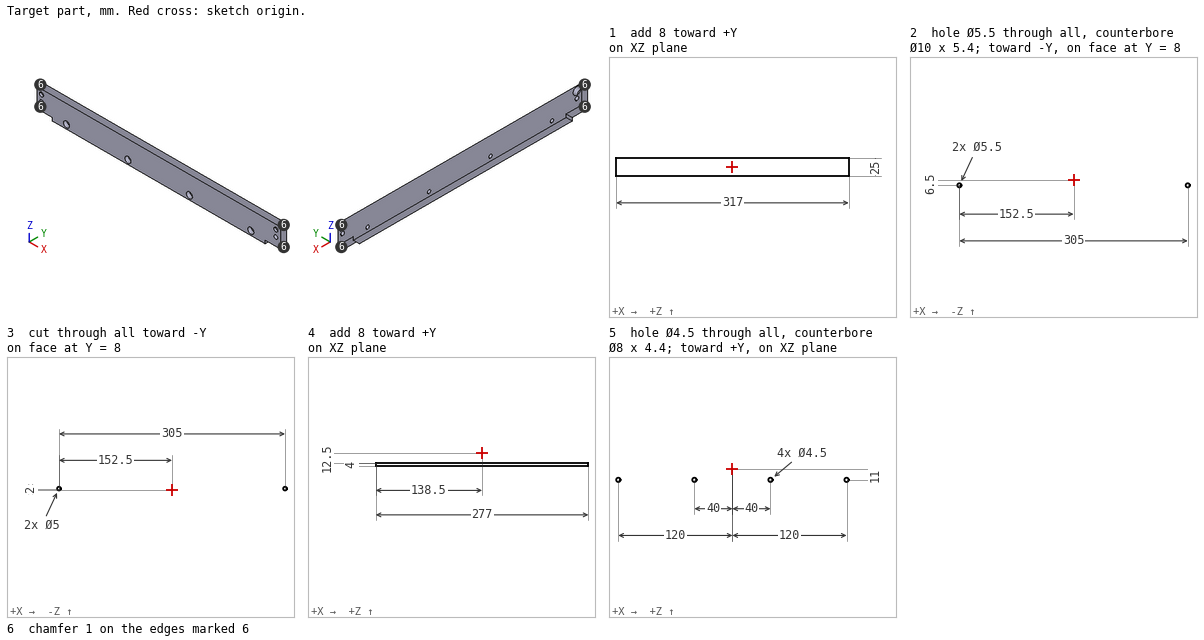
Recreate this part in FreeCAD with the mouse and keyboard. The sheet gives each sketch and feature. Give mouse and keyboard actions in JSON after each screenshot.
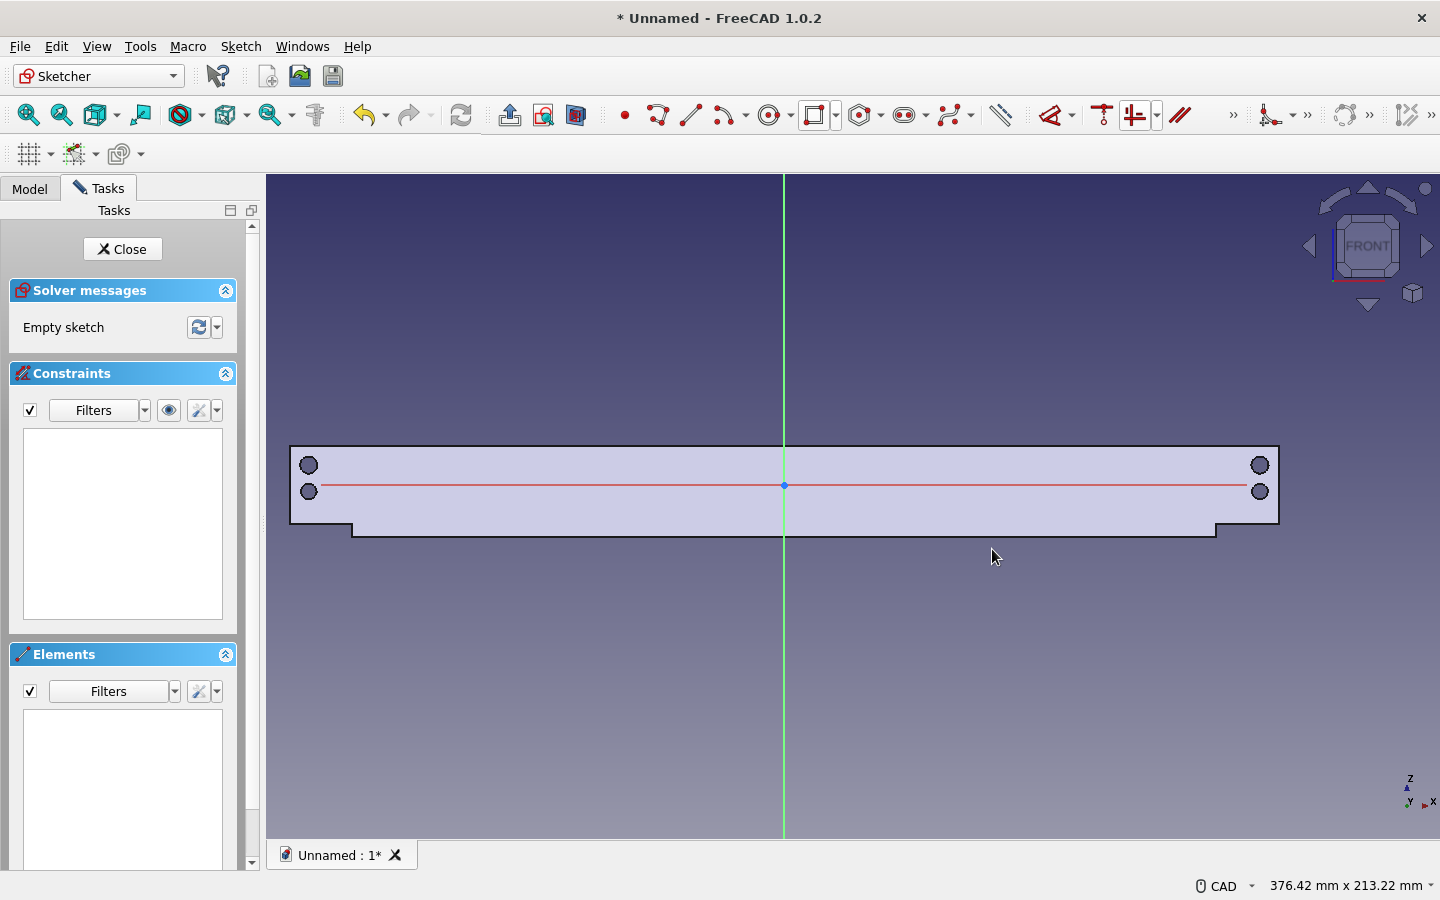
{"action": "left_click", "coordinate": [768, 116]}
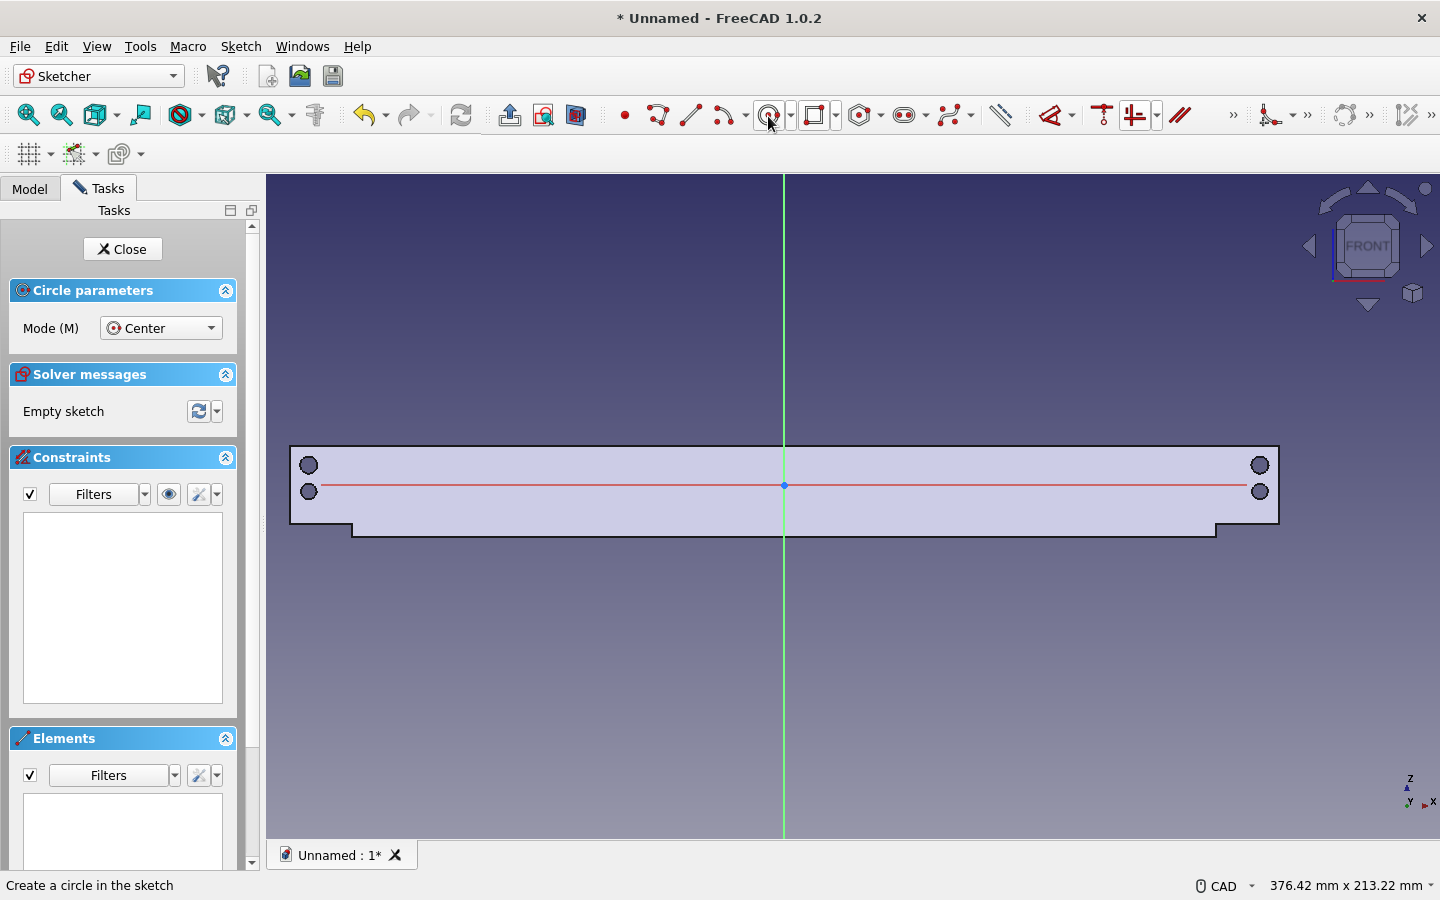
{"action": "scroll", "coordinate": [1159, 520], "scroll_direction": "up", "scroll_amount": 6}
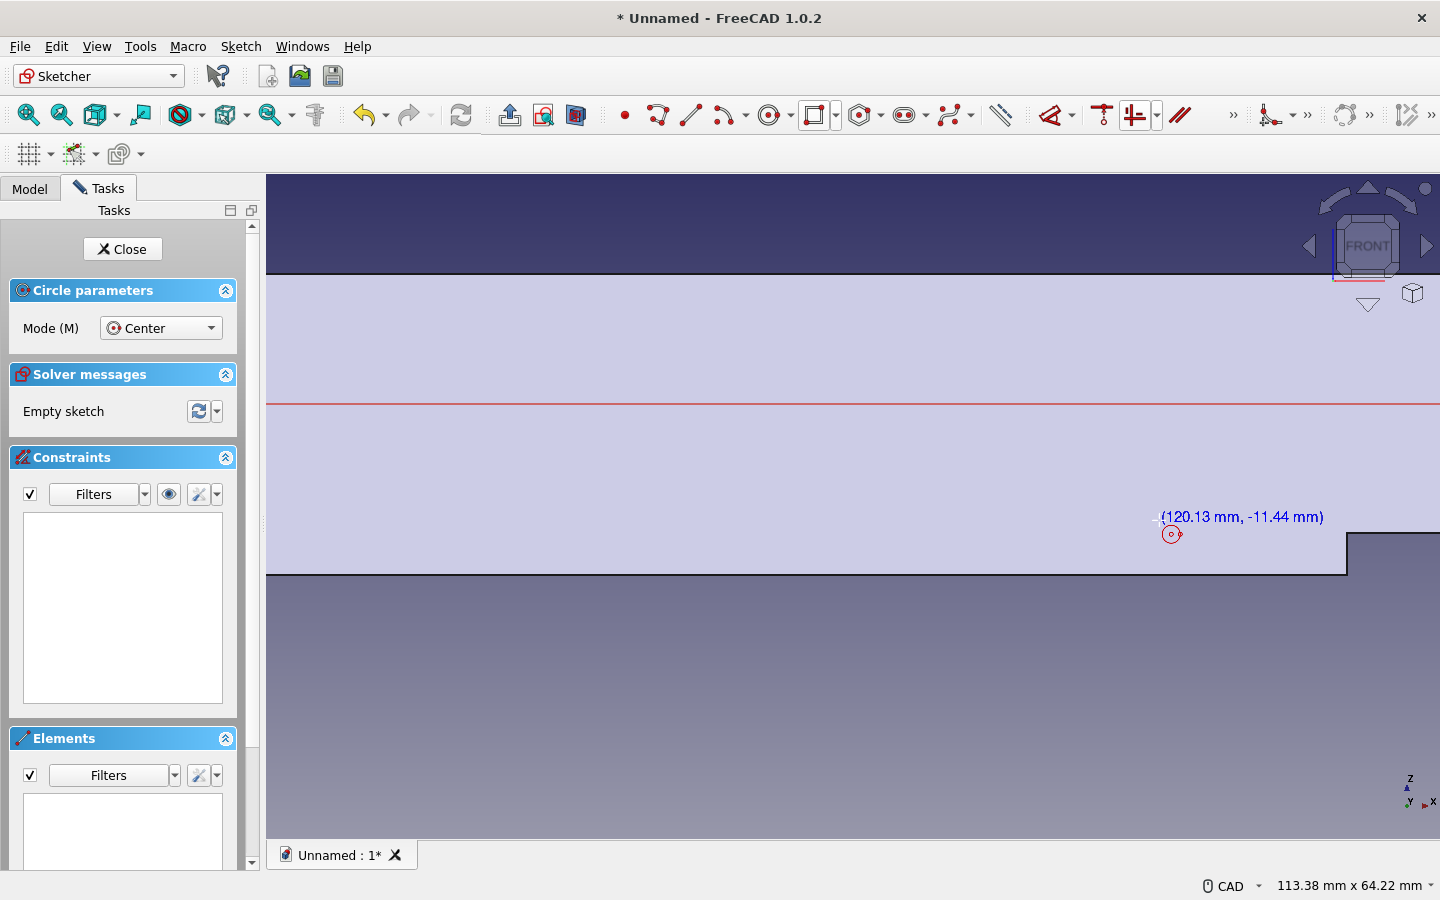
{"action": "left_click", "coordinate": [1156, 518]}
{"action": "mouse_move", "coordinate": [1172, 501]}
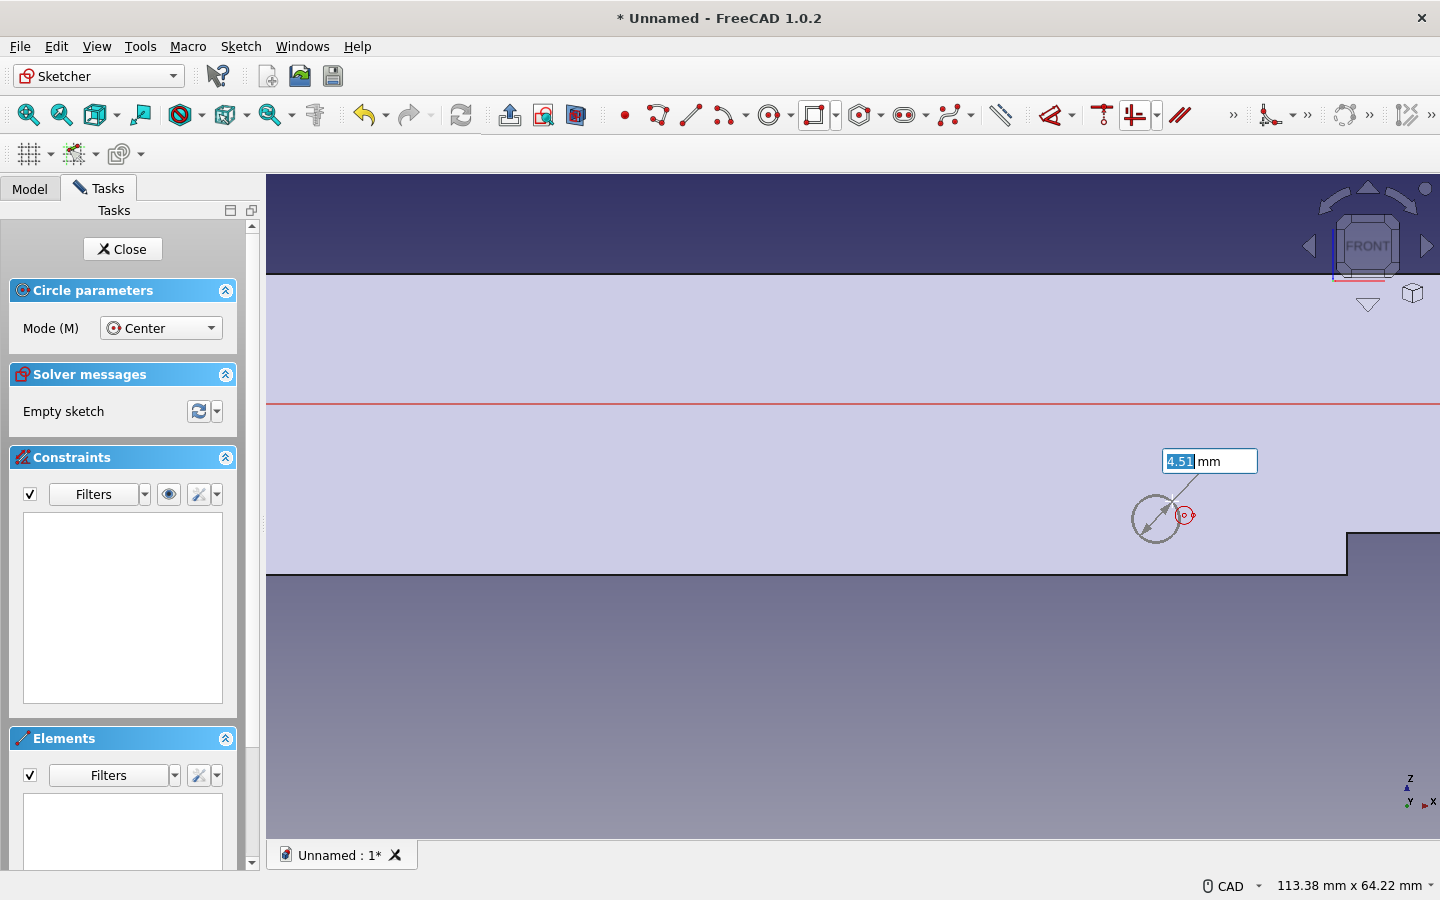
{"action": "type", "text": "4.5"}
{"action": "key", "text": "Return"}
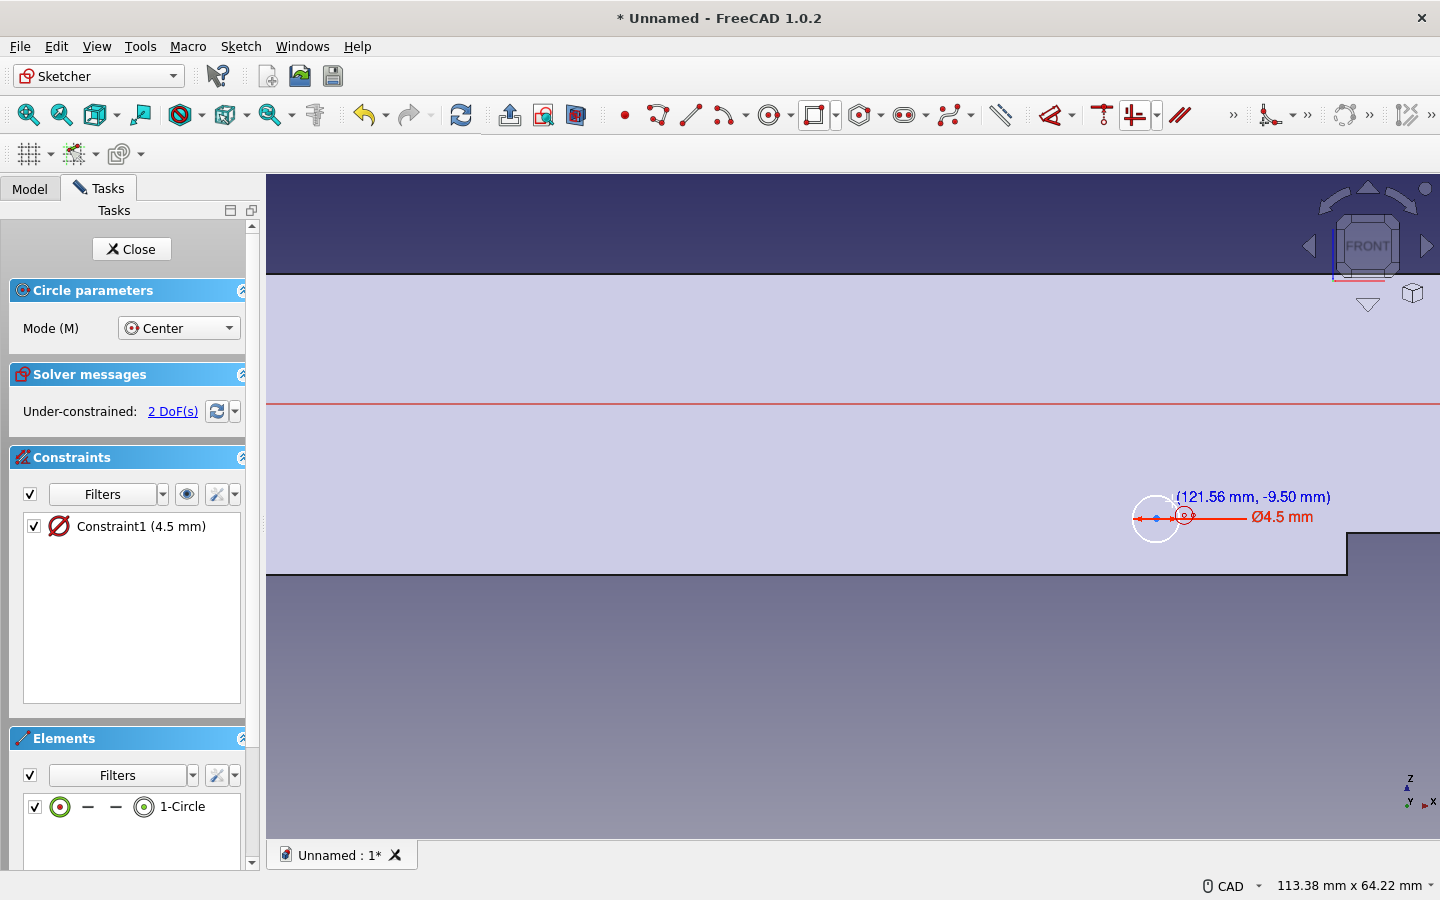
{"action": "left_click", "coordinate": [327, 518]}
{"action": "mouse_move", "coordinate": [344, 501]}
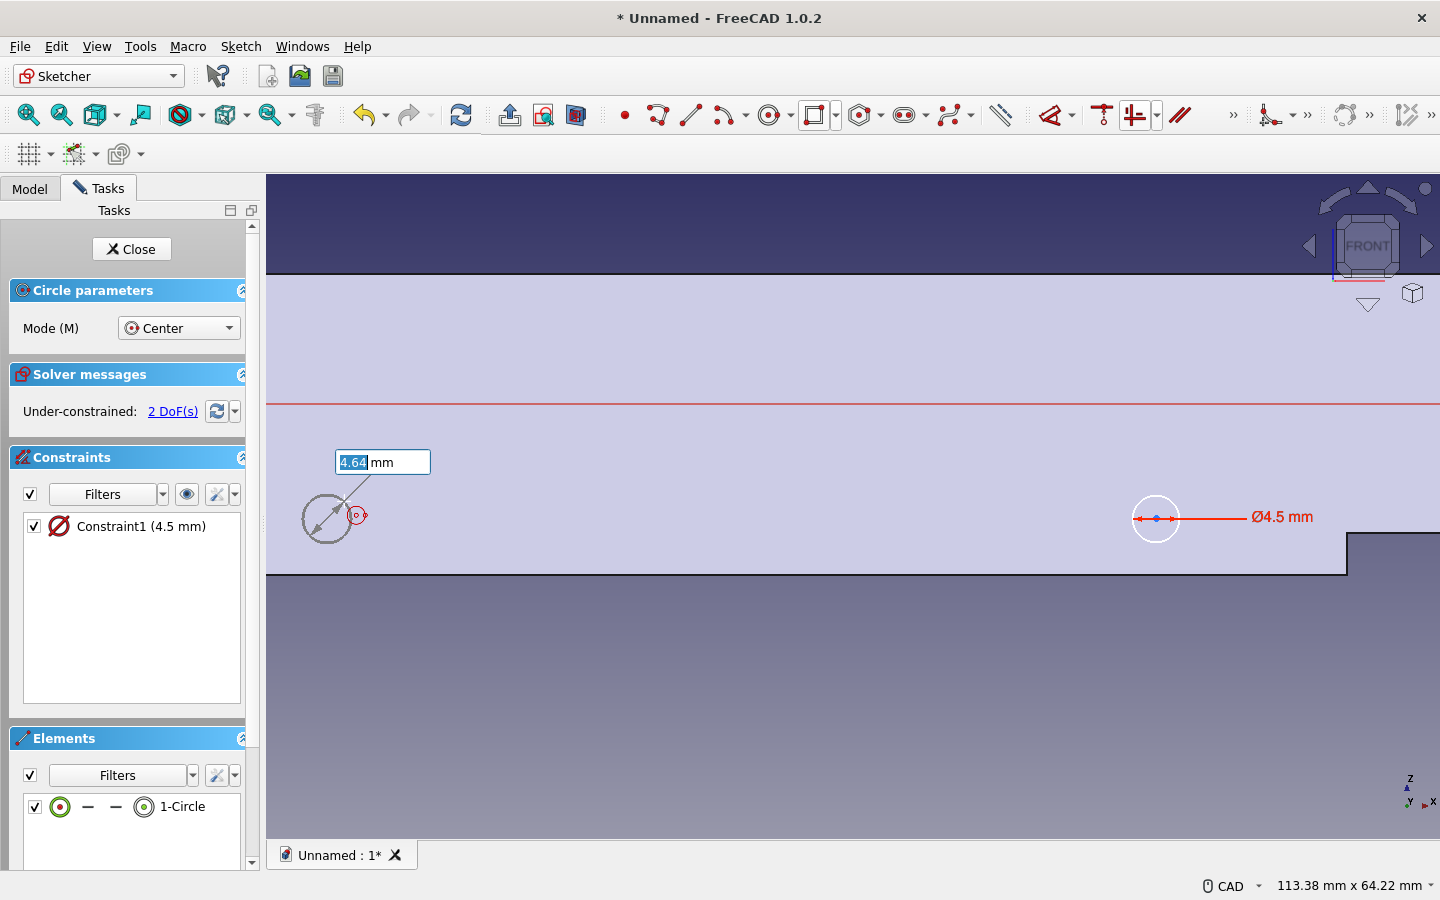
{"action": "type", "text": "4.5"}
{"action": "key", "text": "Return"}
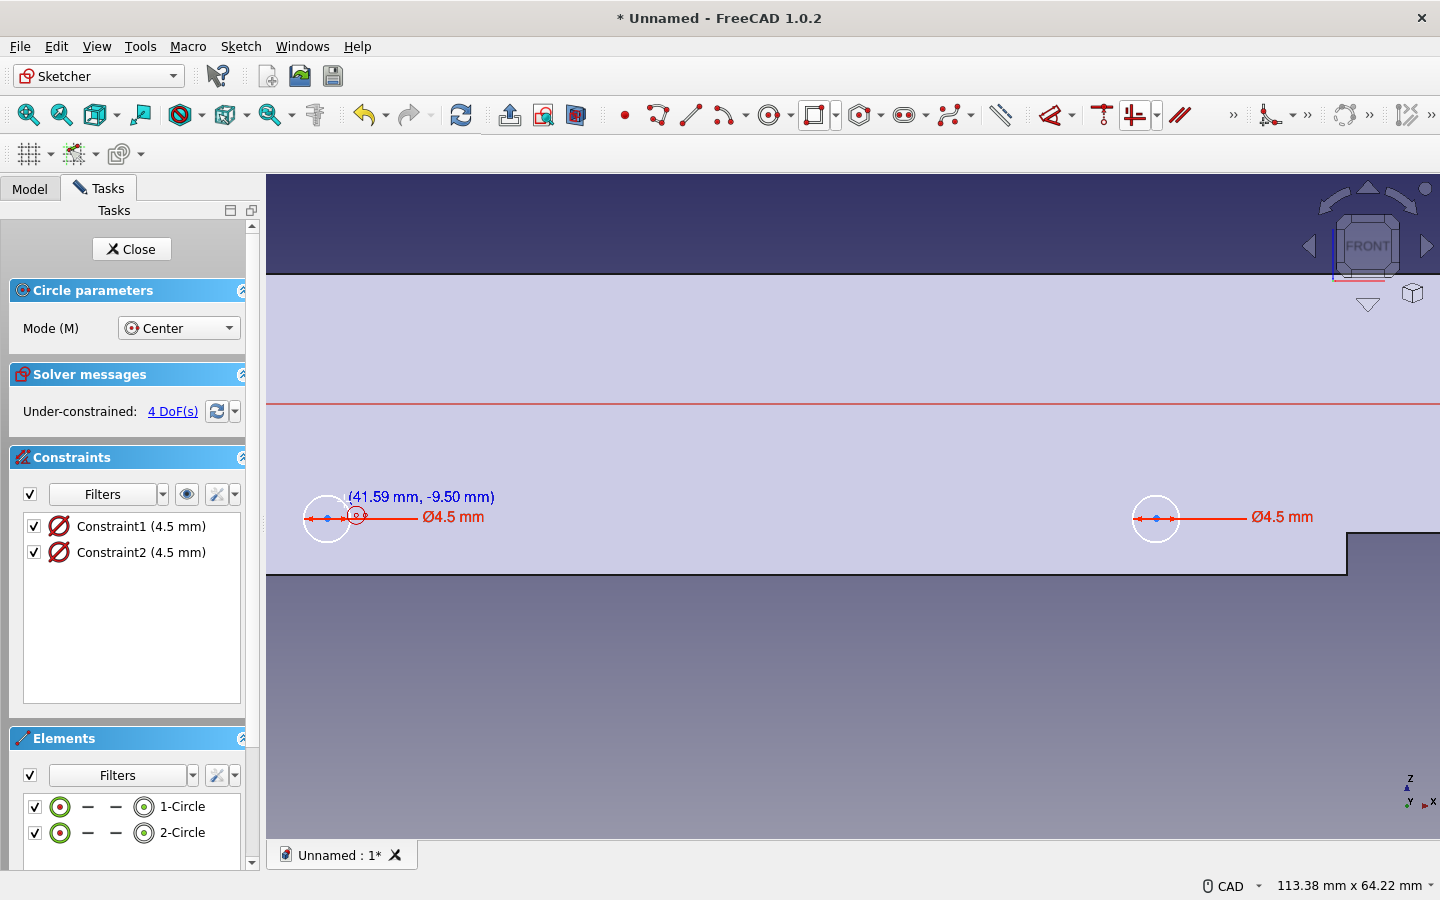
{"action": "scroll", "coordinate": [1160, 521], "scroll_direction": "down", "scroll_amount": 6}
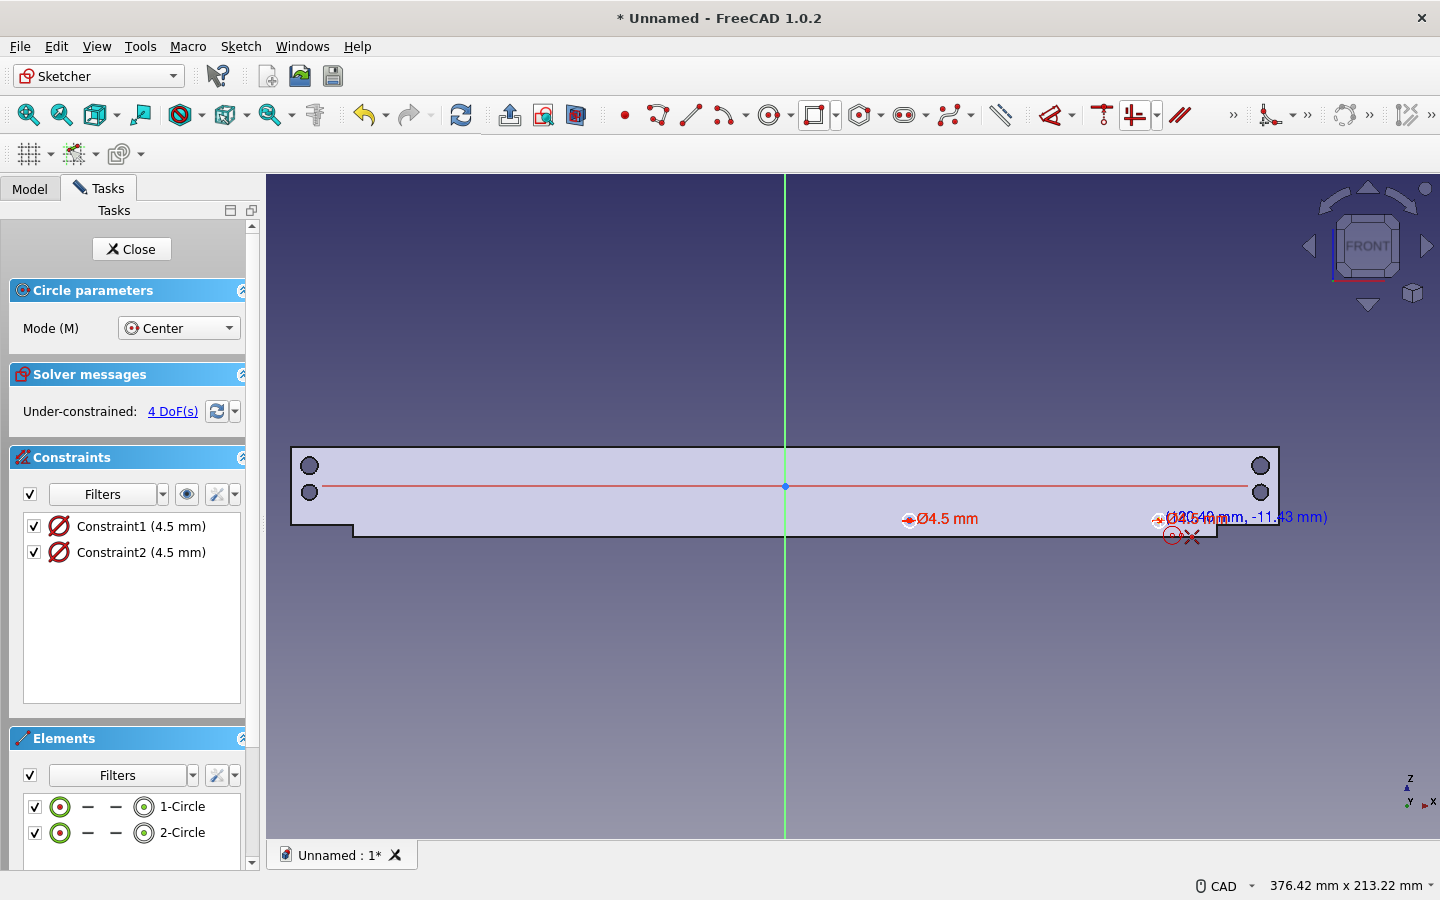
{"action": "scroll", "coordinate": [660, 520], "scroll_direction": "up", "scroll_amount": 6}